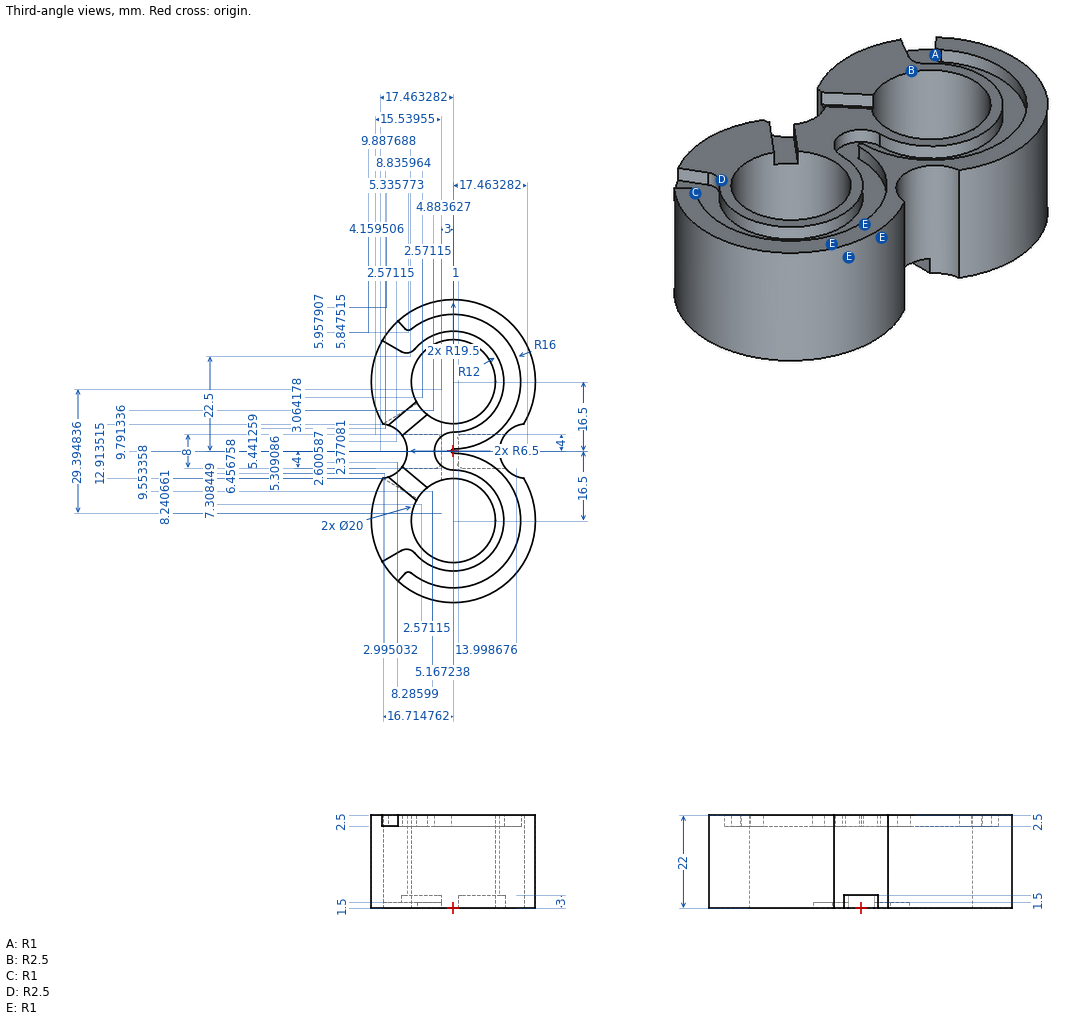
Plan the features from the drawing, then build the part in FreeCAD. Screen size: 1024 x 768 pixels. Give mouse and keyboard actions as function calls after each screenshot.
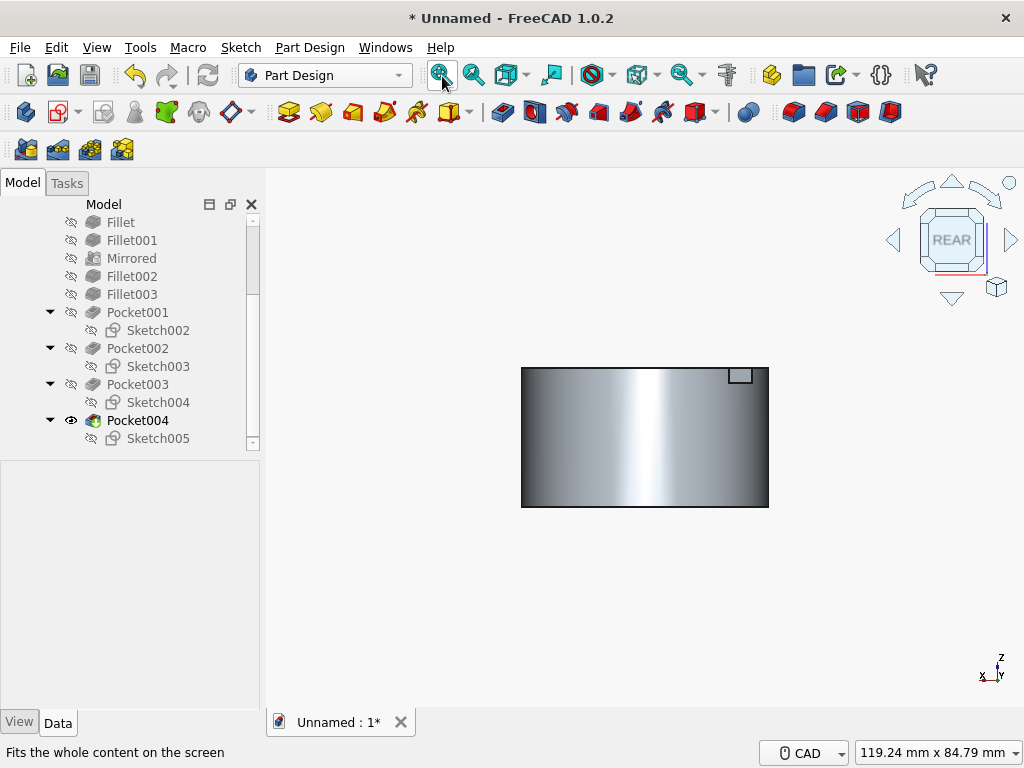
key(v)
key(f)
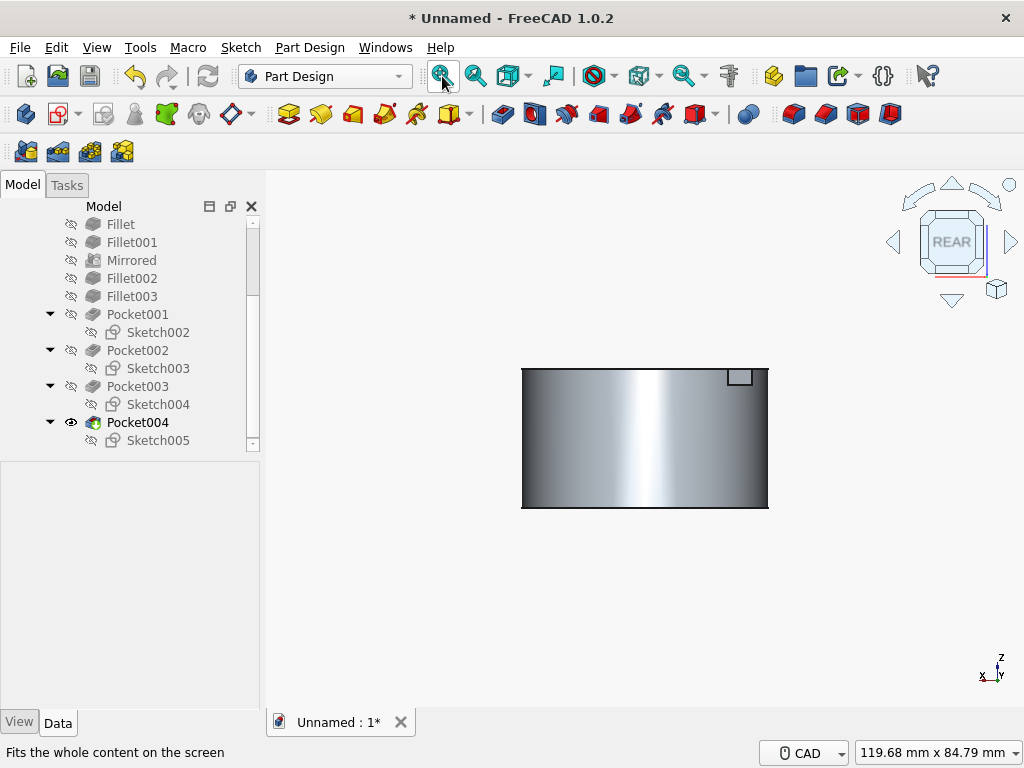
scroll(664, 493, up, 8)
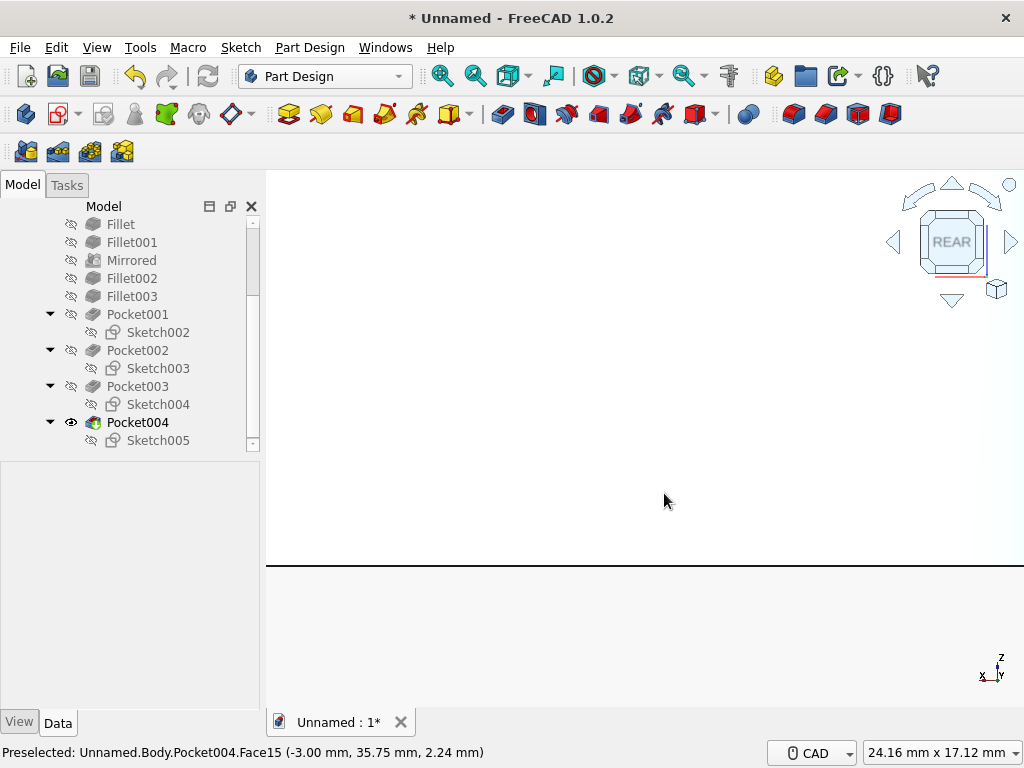
key(v)
key(f)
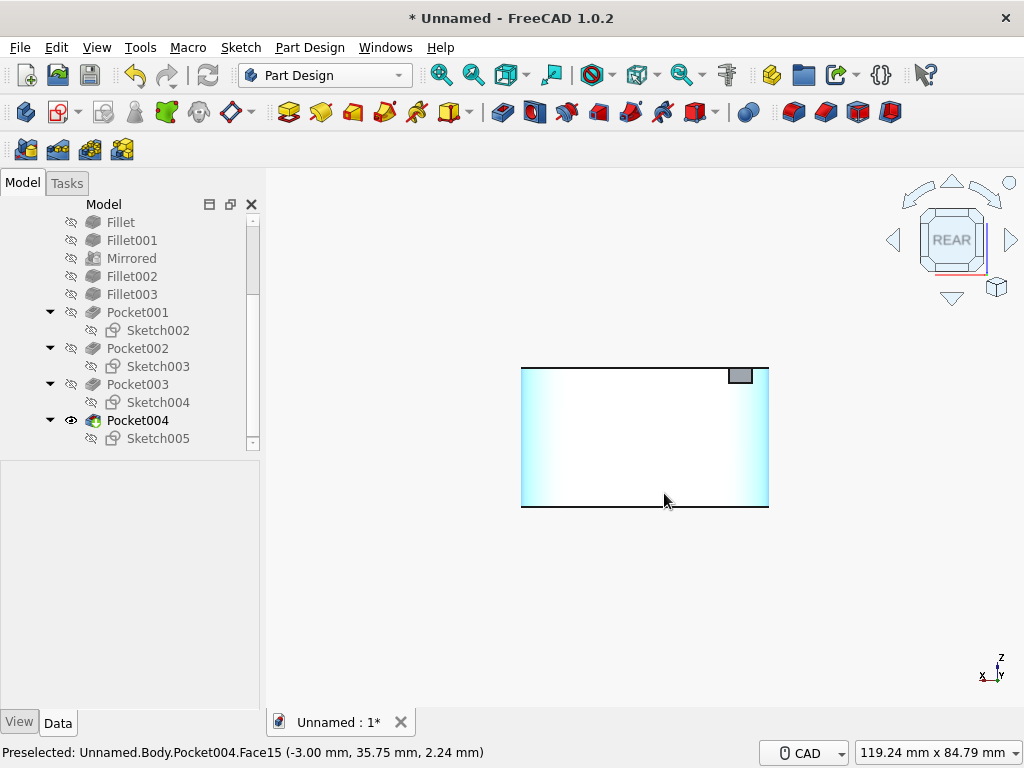
key(6)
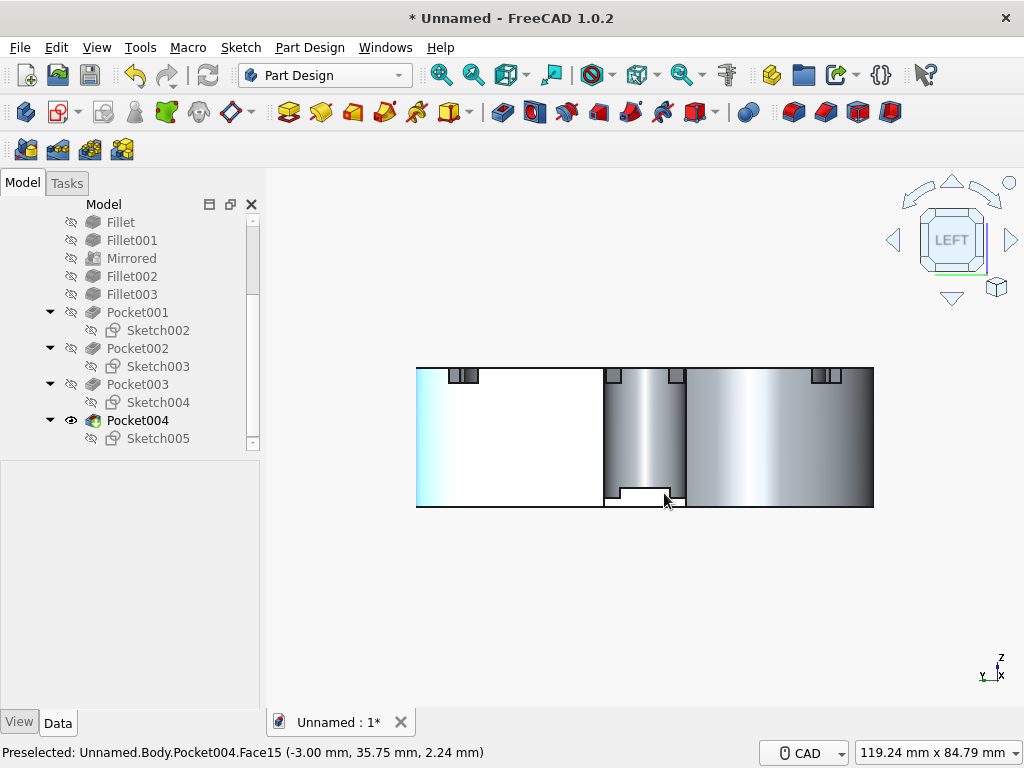
scroll(620, 492, up, 8)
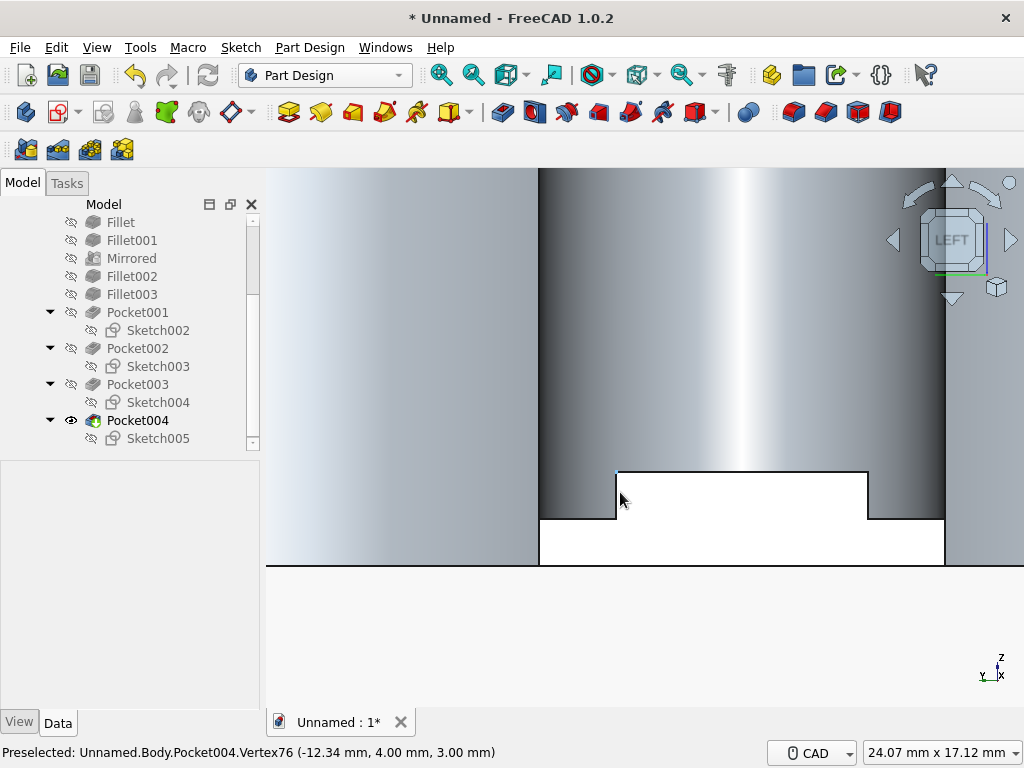
click(442, 76)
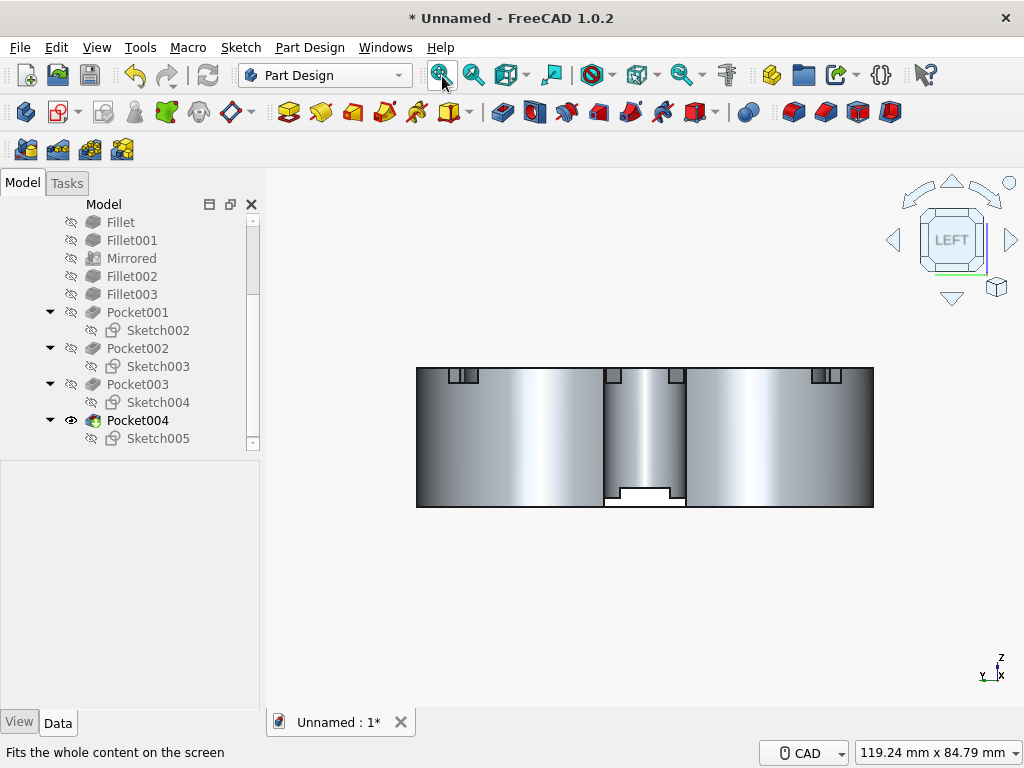
key(v)
key(3)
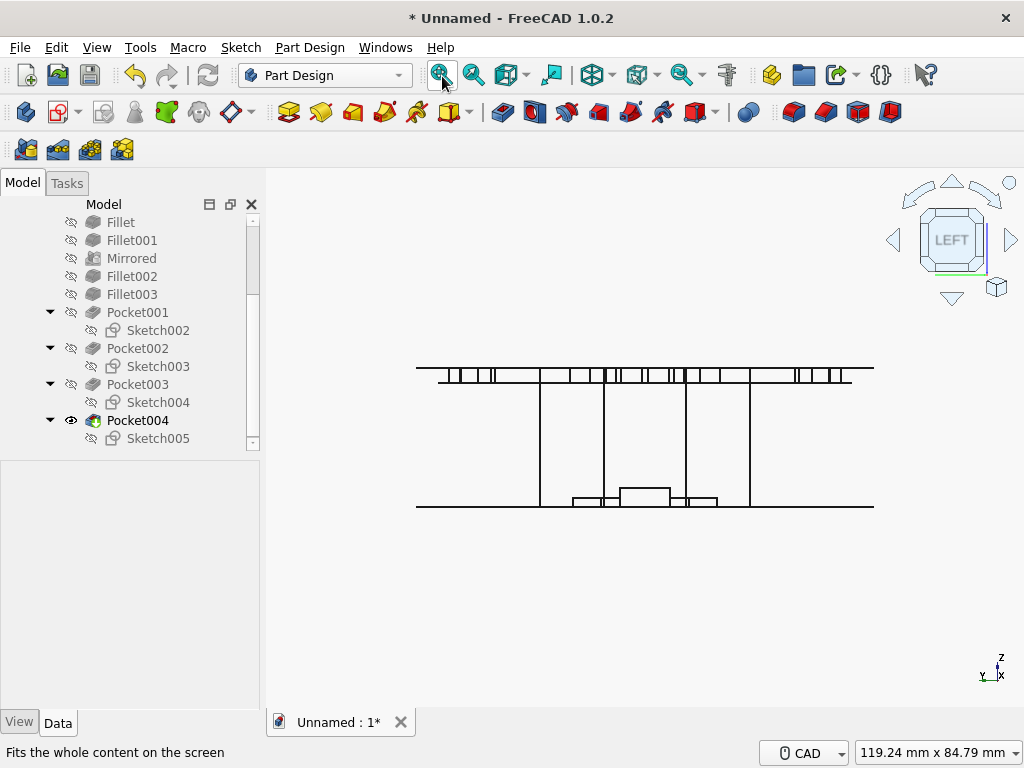
key(0)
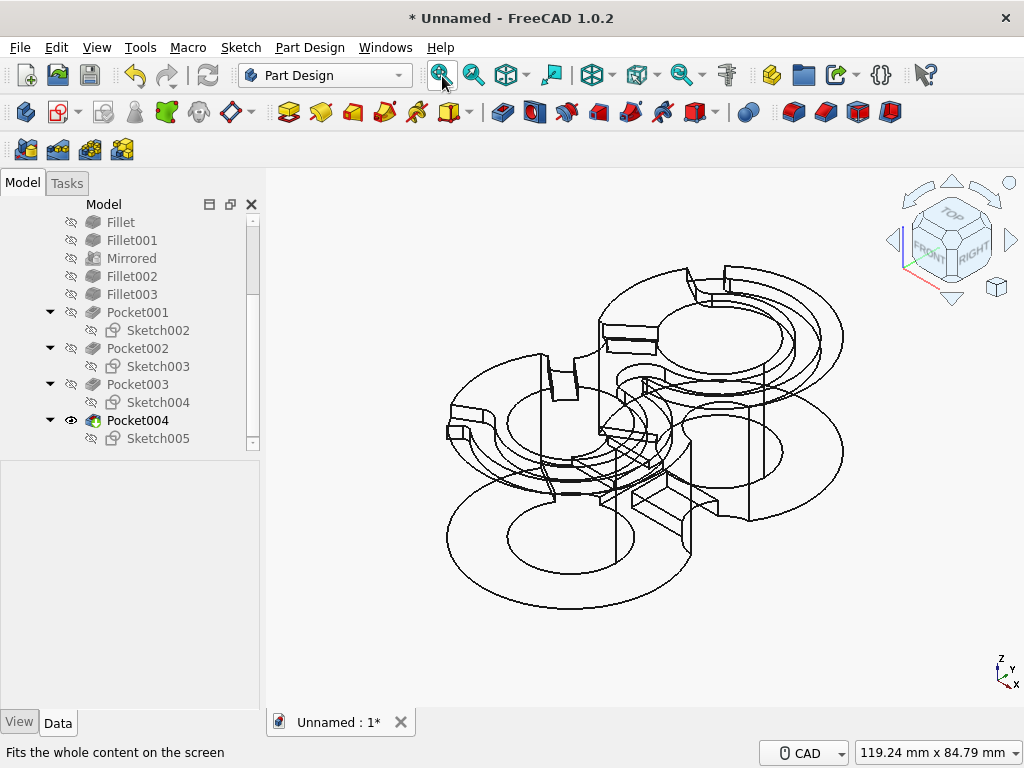
click(667, 478)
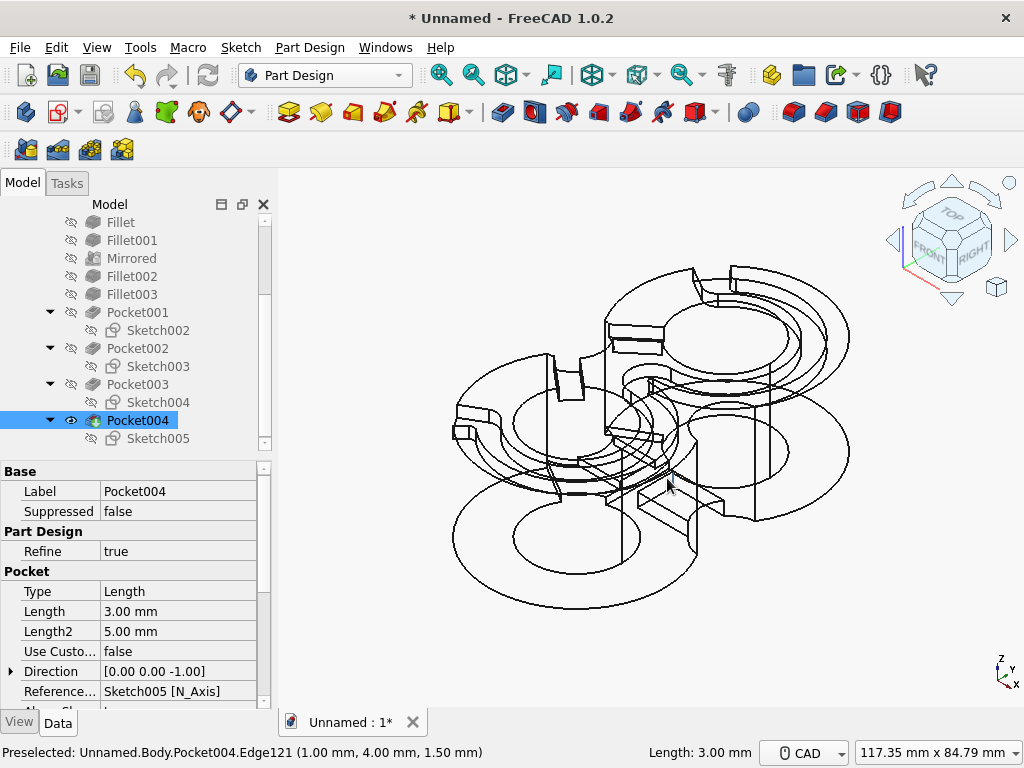
click(638, 499, ctrl)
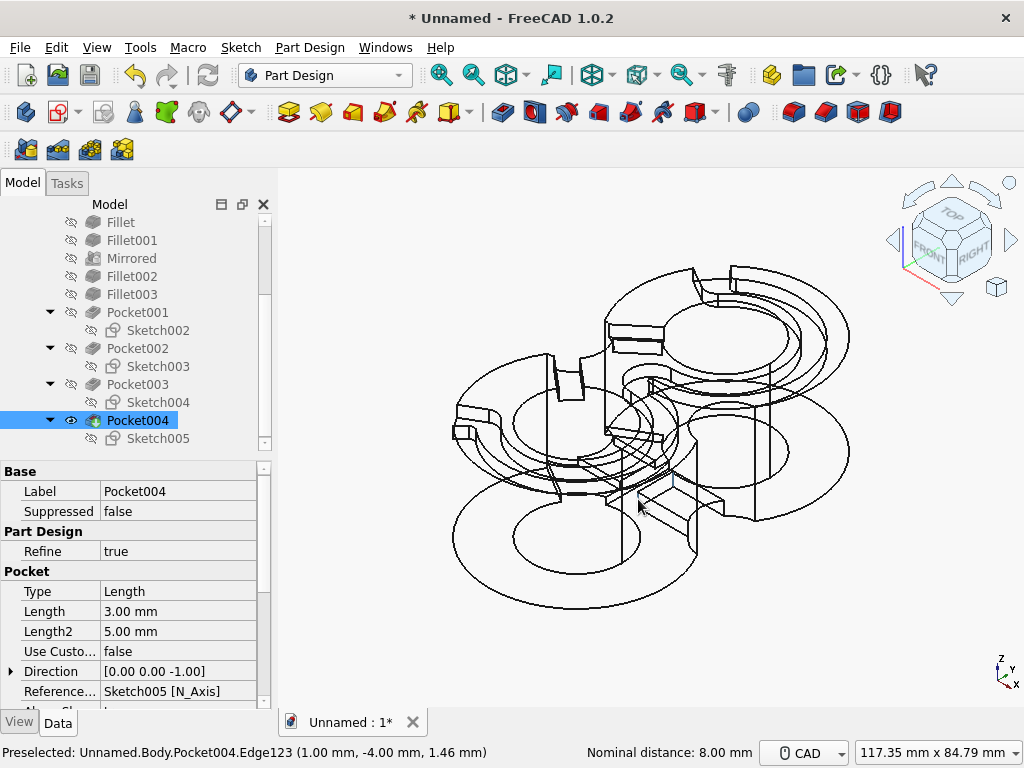
scroll(655, 464, up, 8)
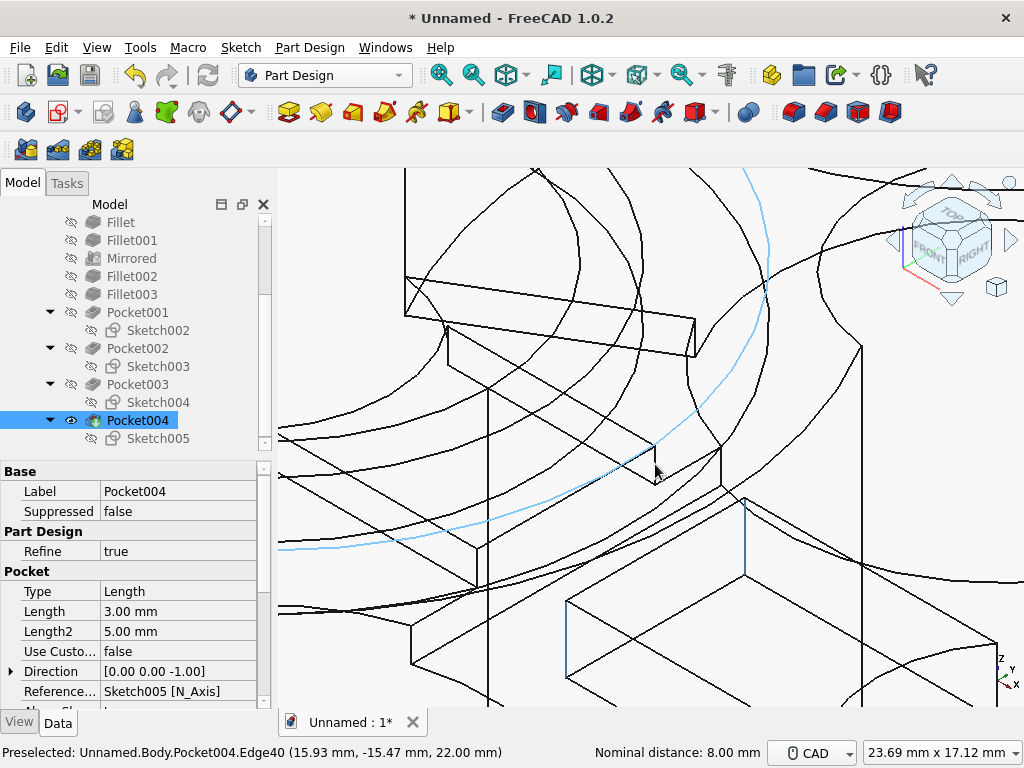
click(655, 465, ctrl)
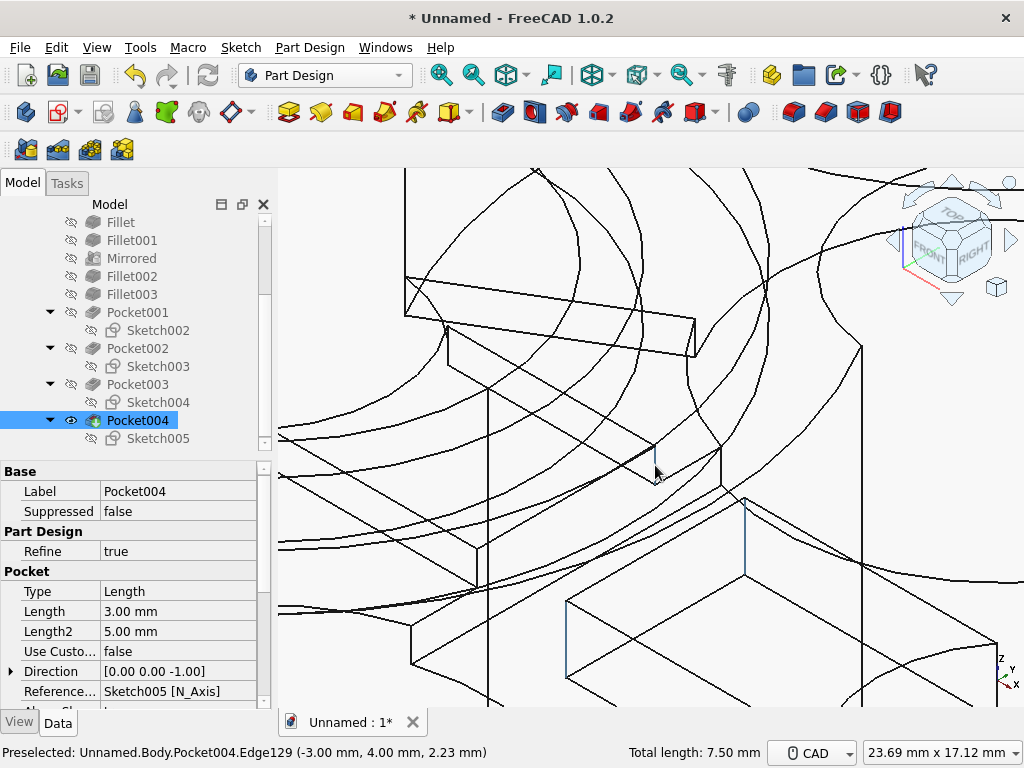
click(477, 567, ctrl)